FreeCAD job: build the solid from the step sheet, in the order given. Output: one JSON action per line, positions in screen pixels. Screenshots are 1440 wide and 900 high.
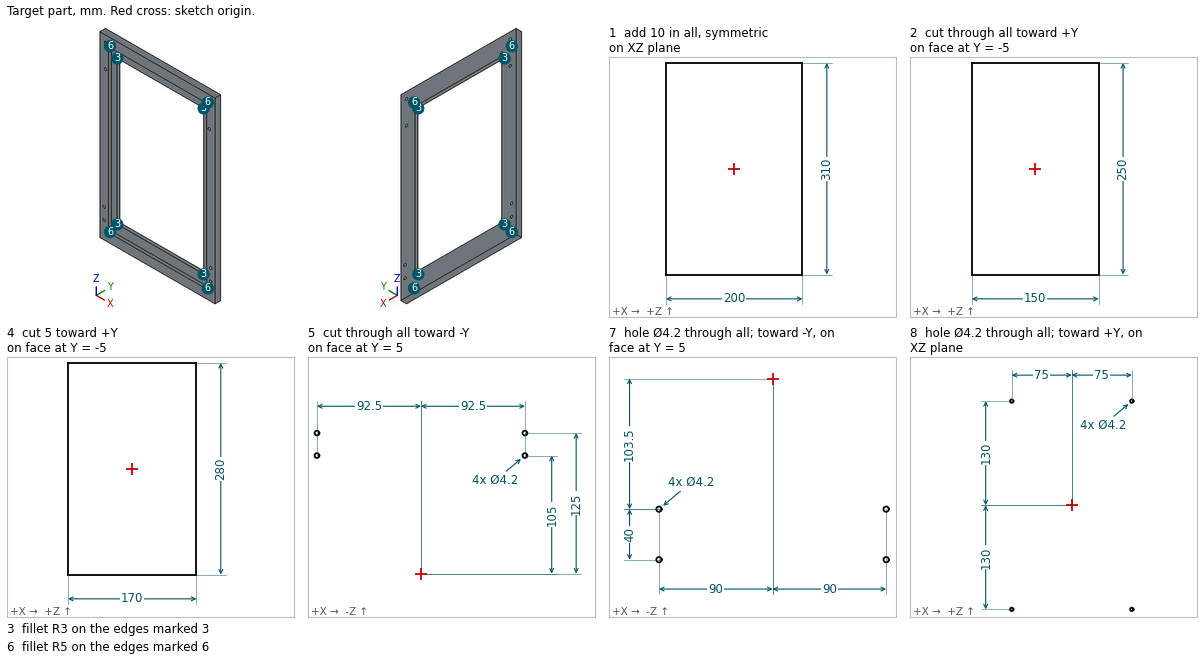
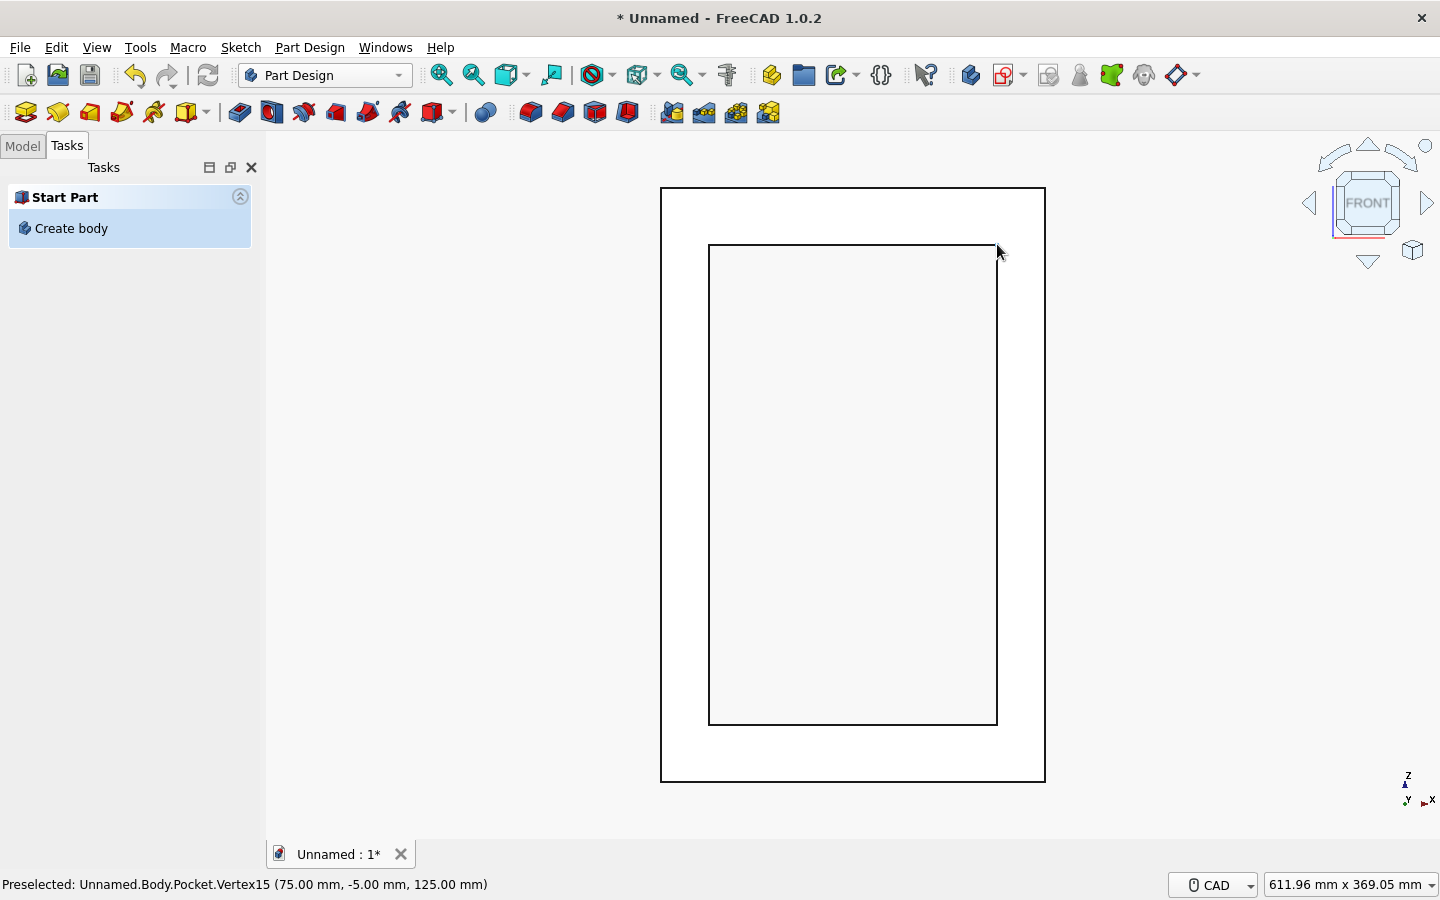
{"action": "key", "text": "3"}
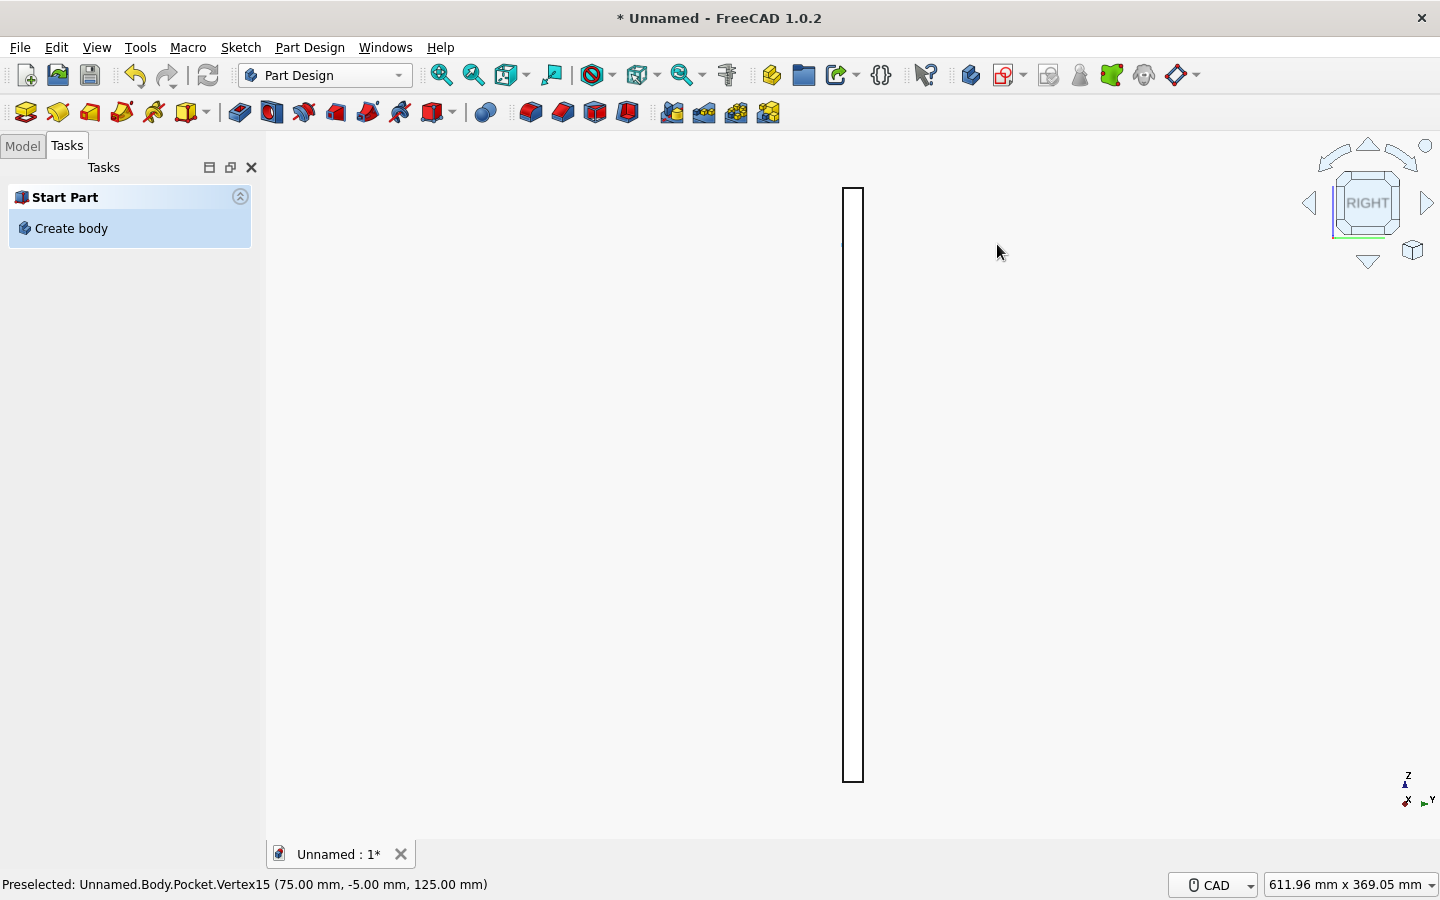
{"action": "scroll", "coordinate": [853, 244], "scroll_direction": "up", "scroll_amount": 4}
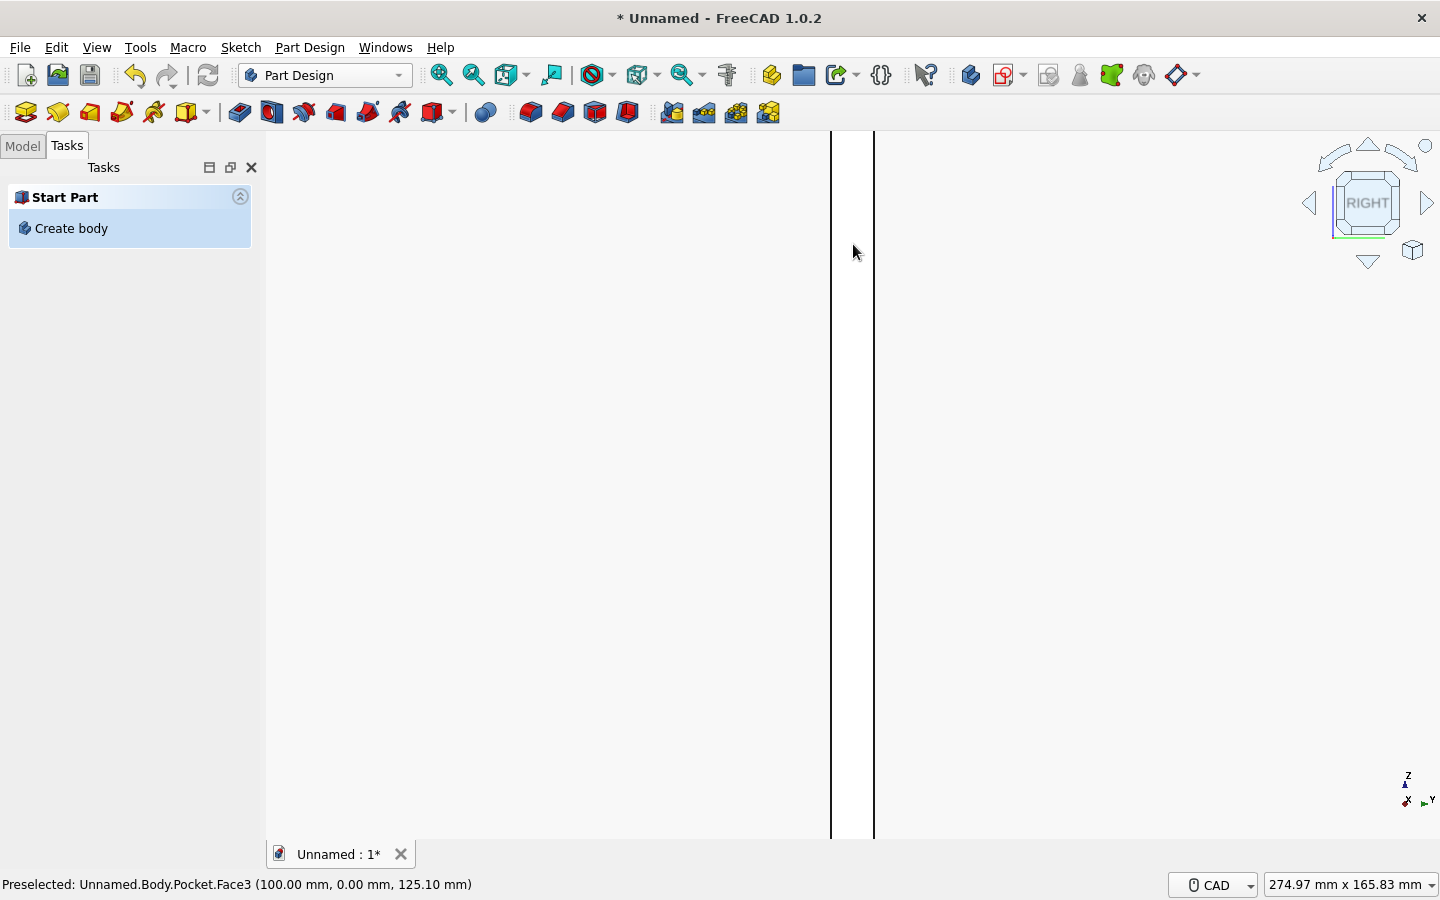
{"action": "key", "text": "v f"}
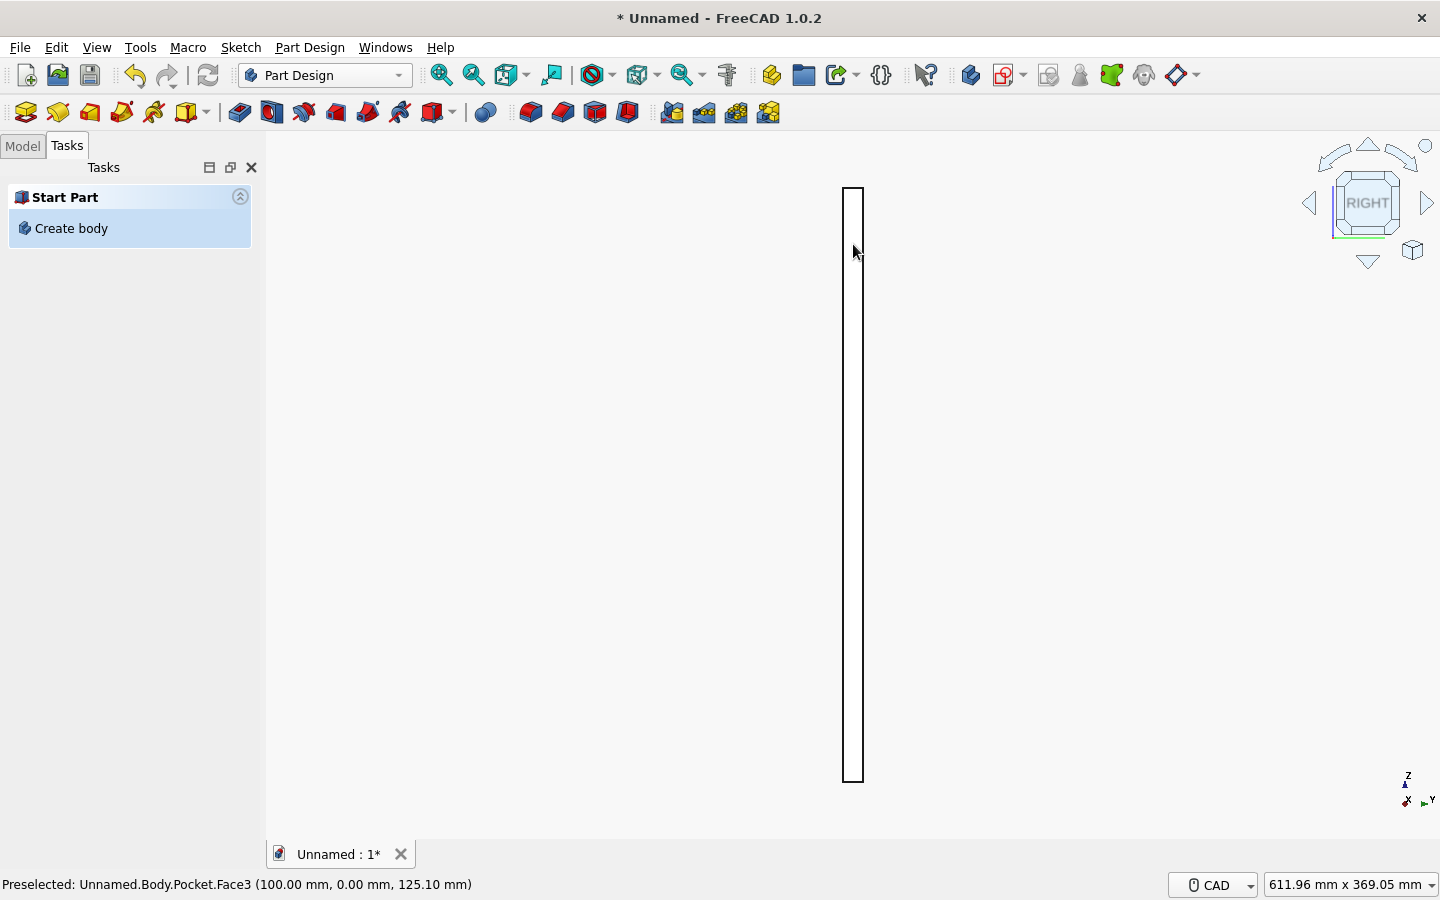
{"action": "key", "text": "5"}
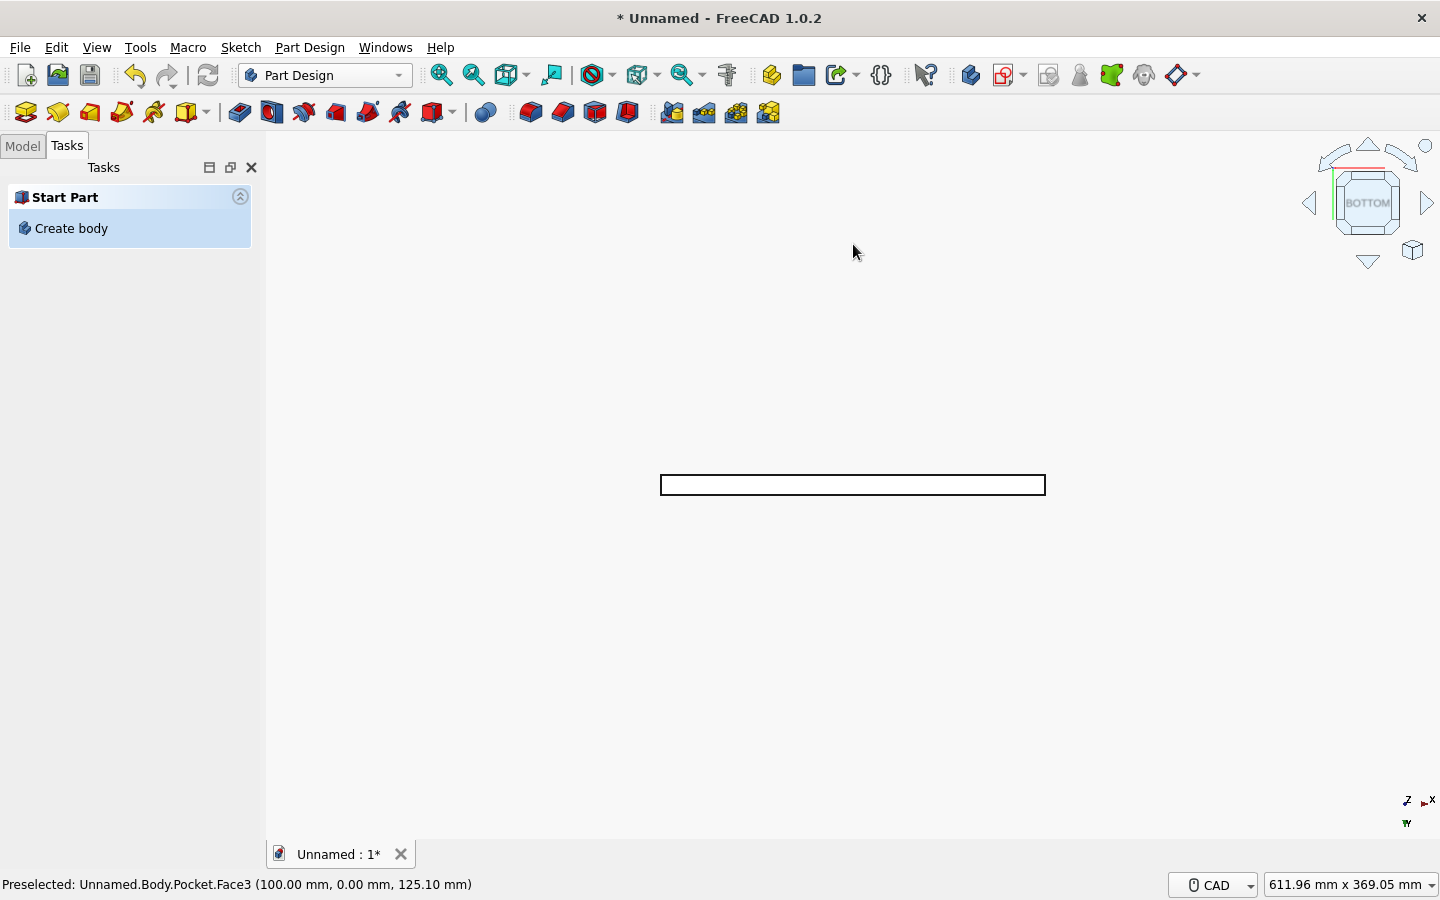
{"action": "left_click", "coordinate": [442, 76]}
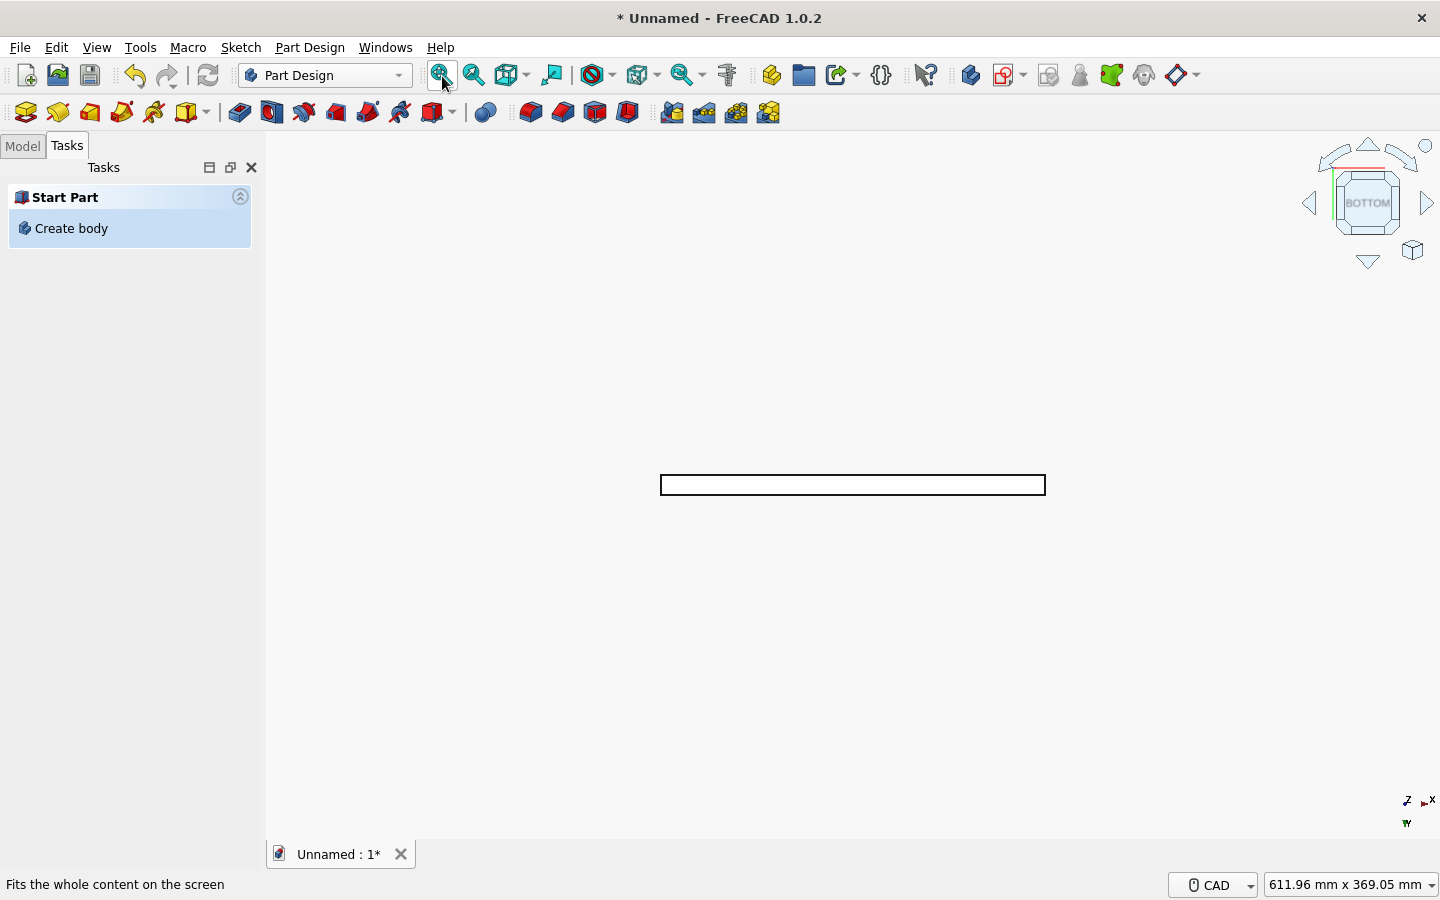
{"action": "scroll", "coordinate": [997, 484], "scroll_direction": "up", "scroll_amount": 4}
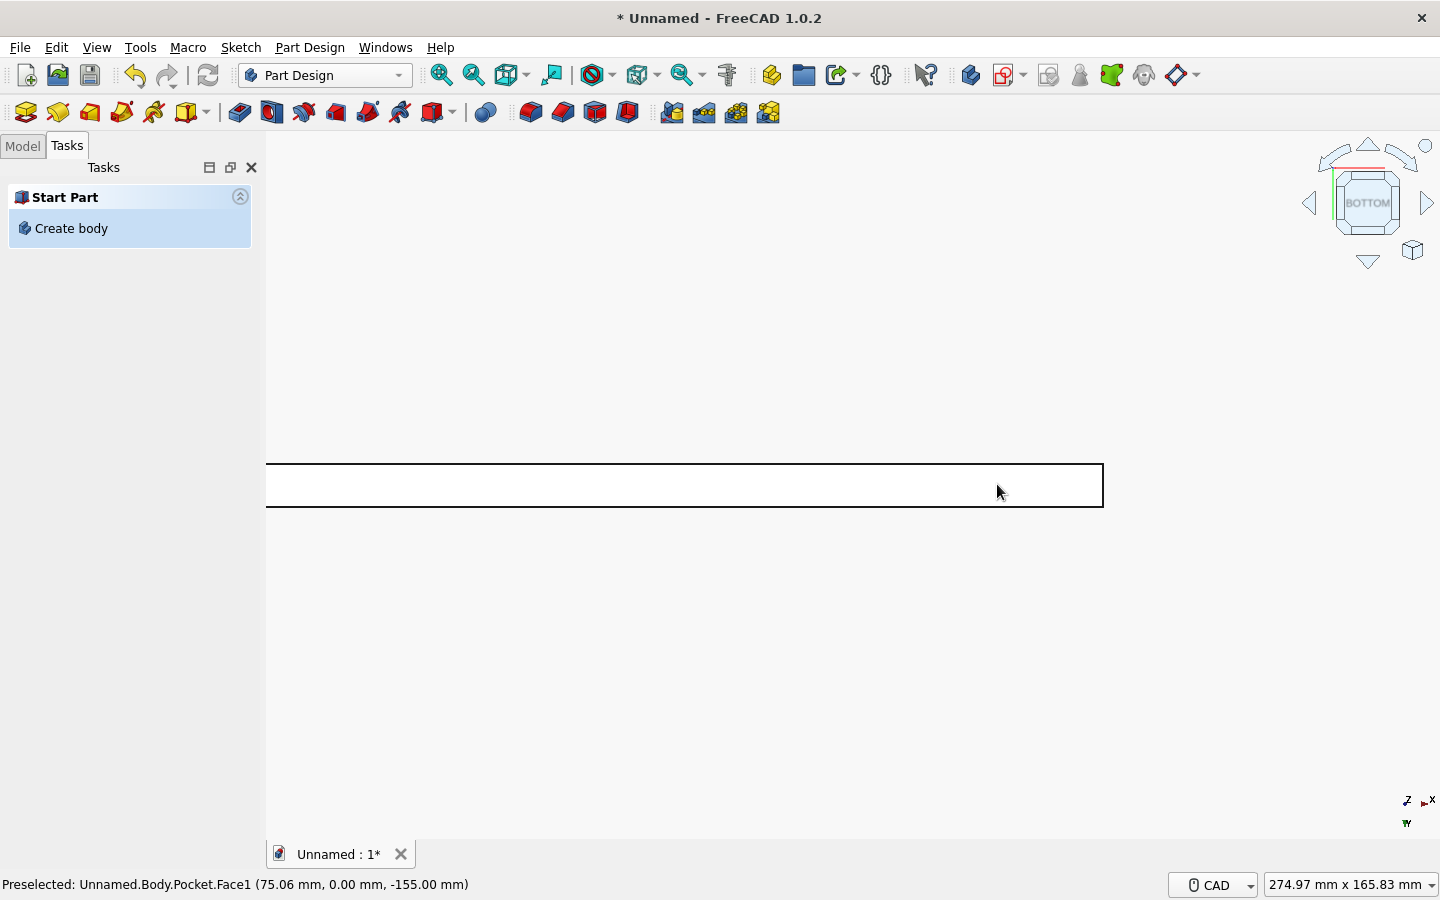
{"action": "key", "text": "v f"}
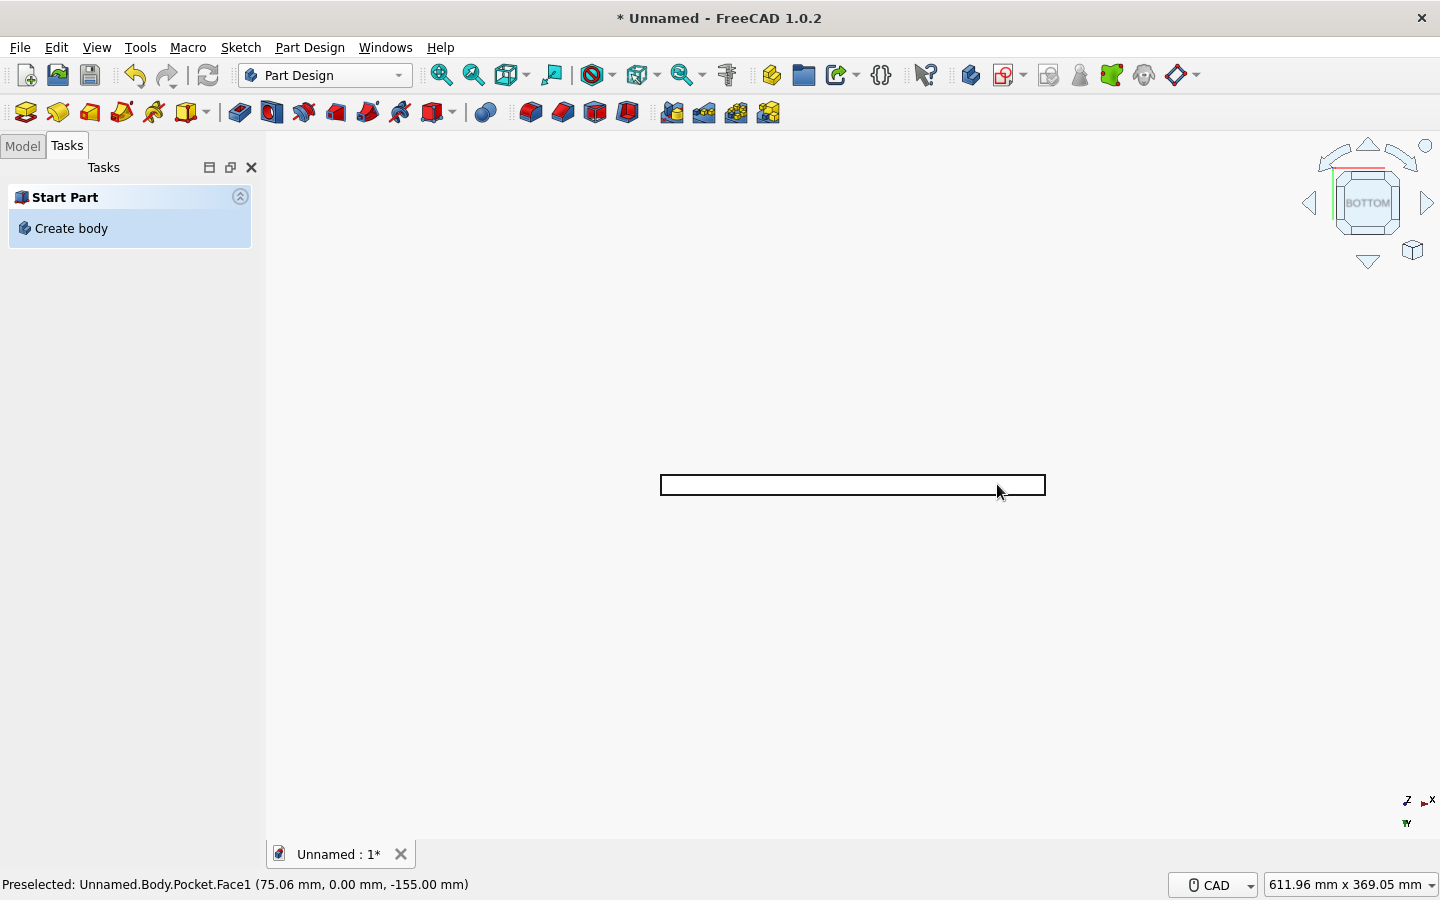
{"action": "key", "text": "4"}